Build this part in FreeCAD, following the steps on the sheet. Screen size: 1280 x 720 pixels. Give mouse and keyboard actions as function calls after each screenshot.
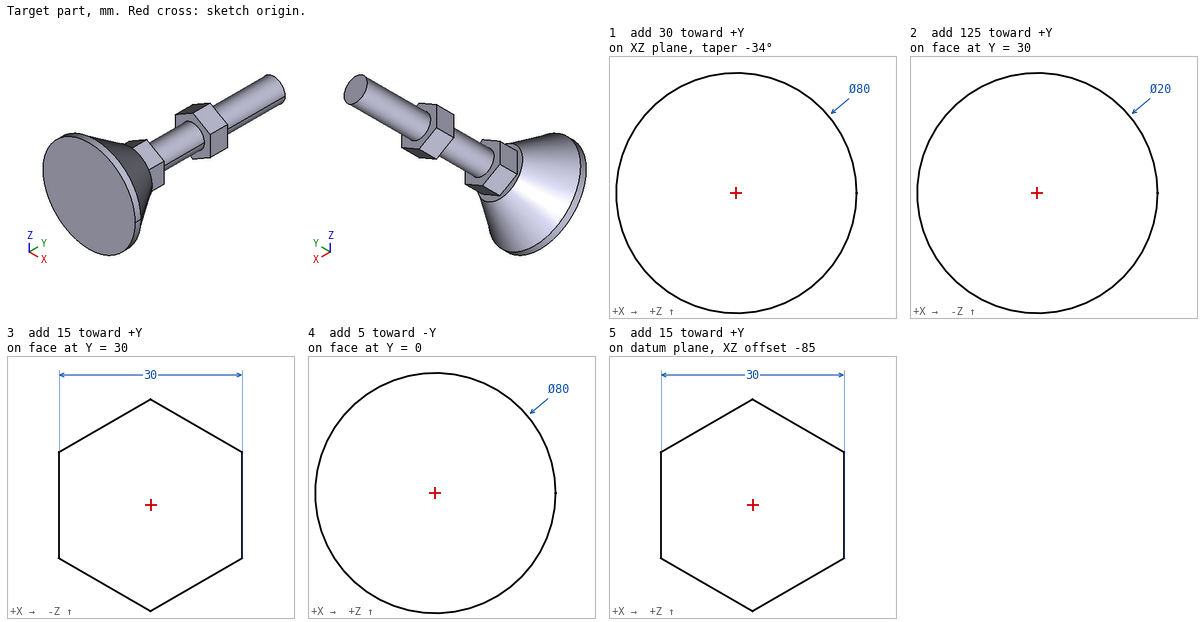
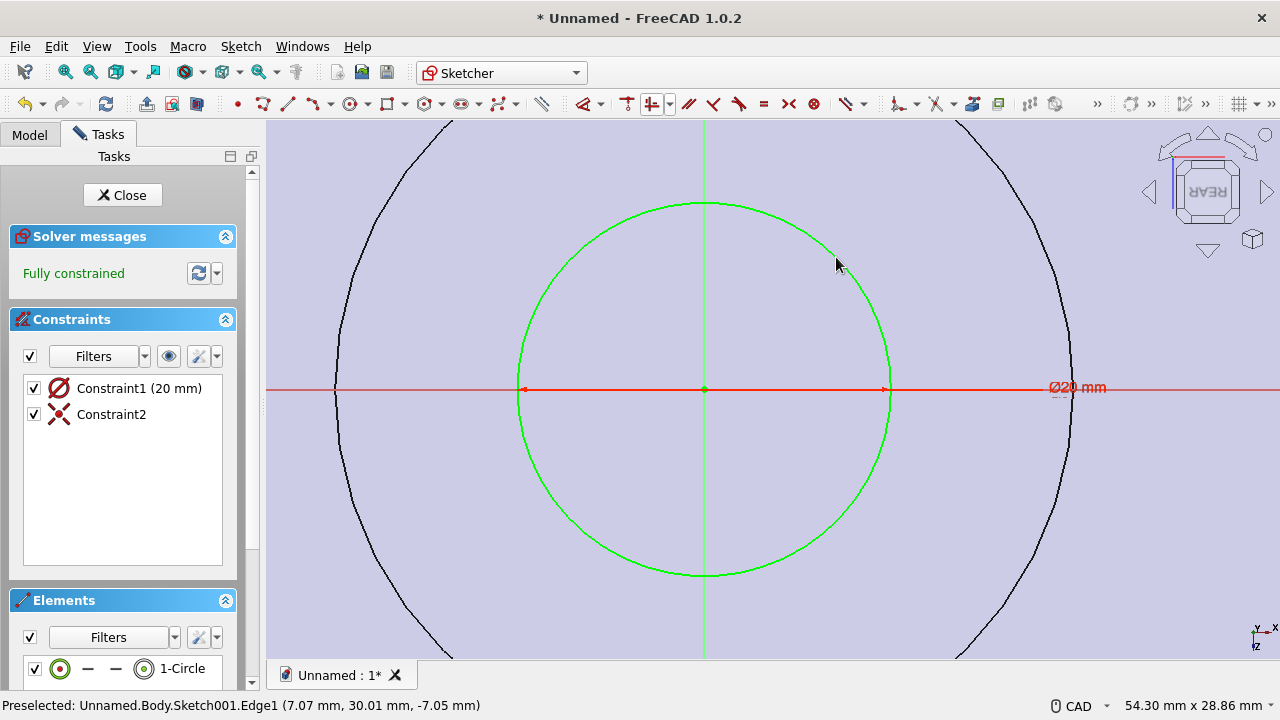
click(123, 195)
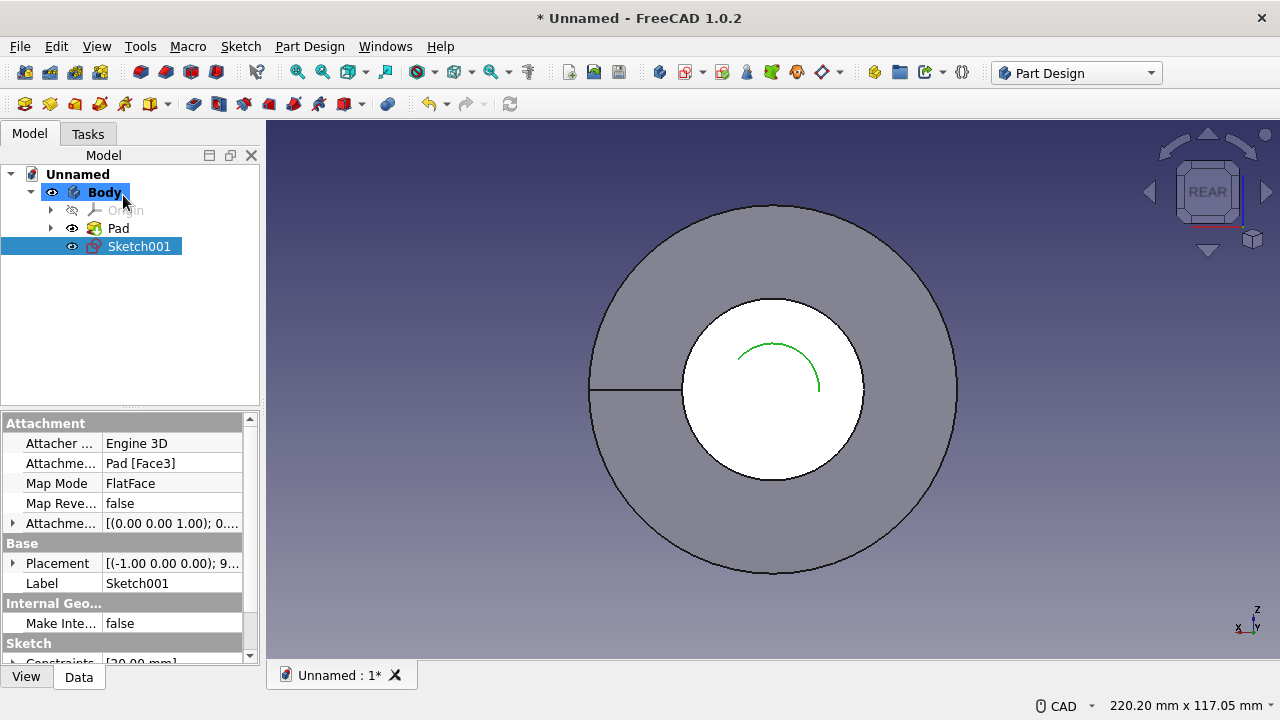
click(25, 104)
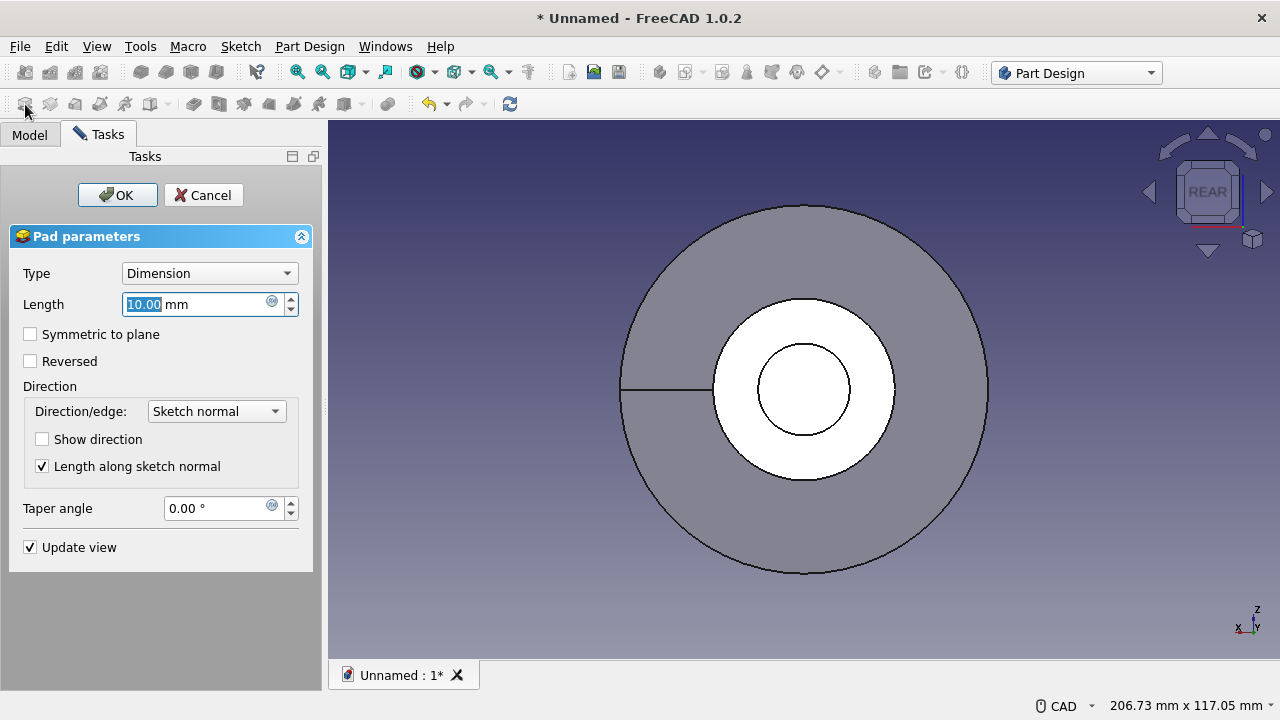
text(125)
key(Tab)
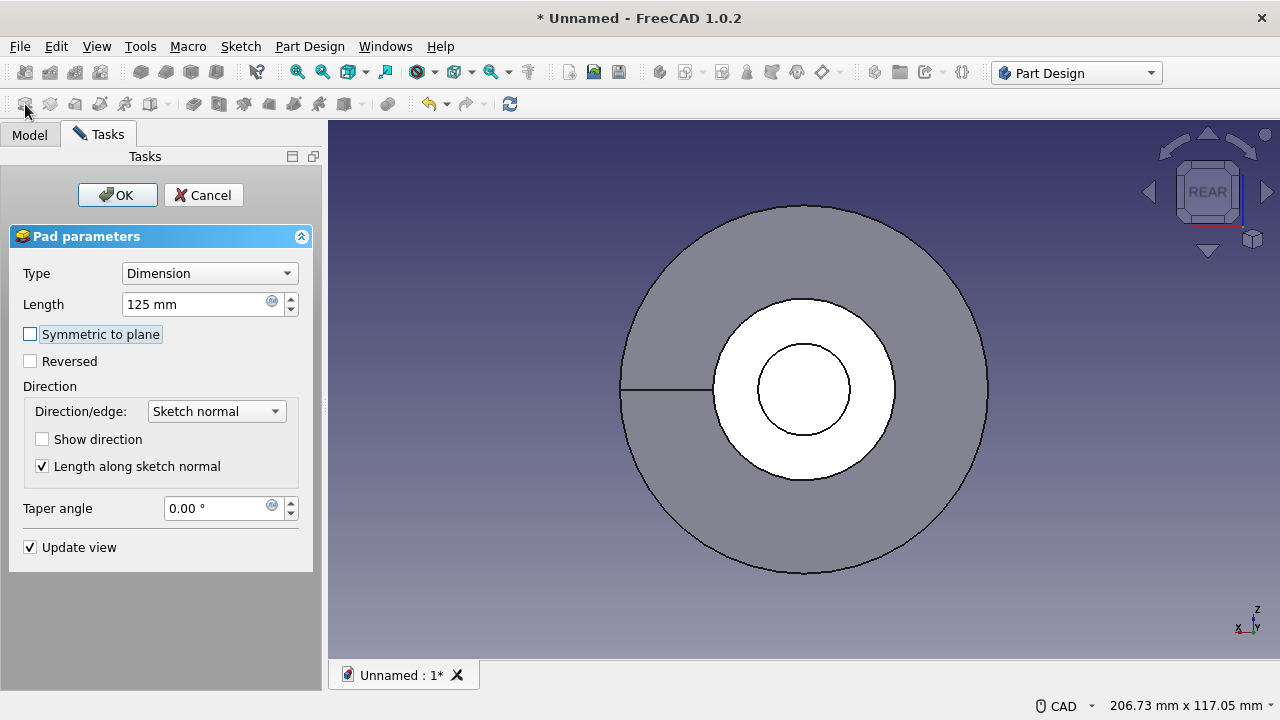
click(118, 195)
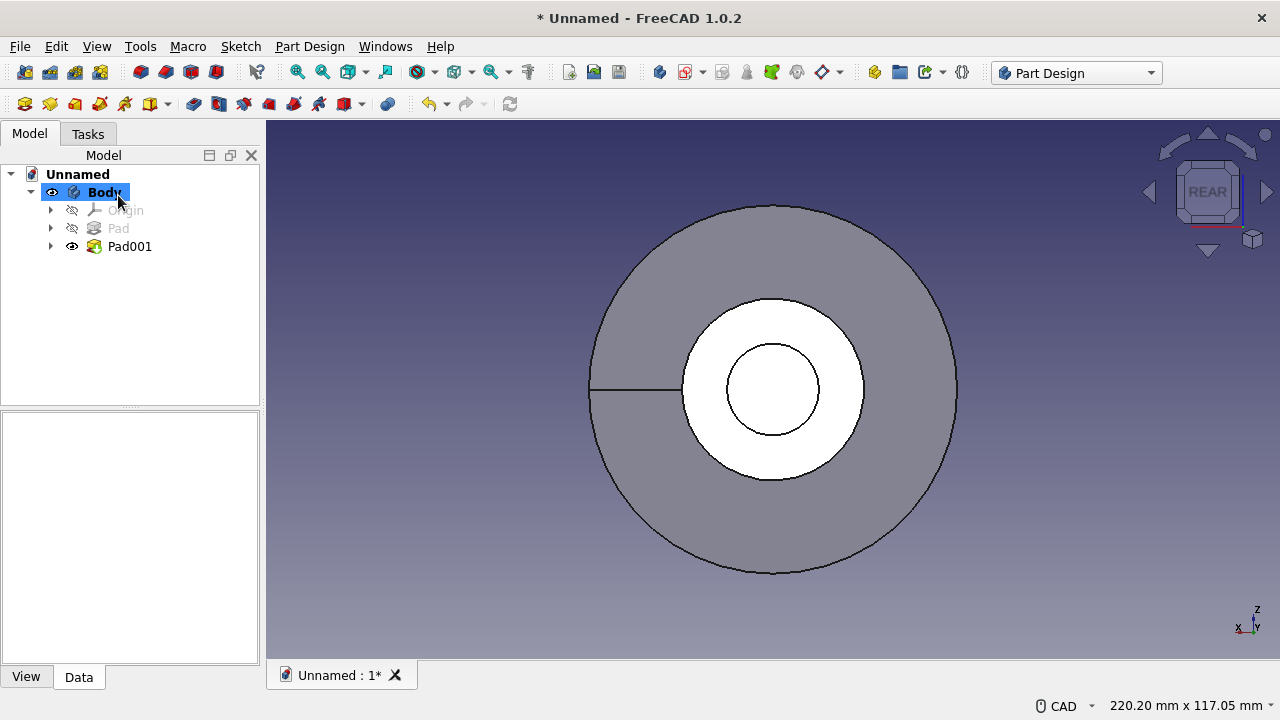
click(721, 336)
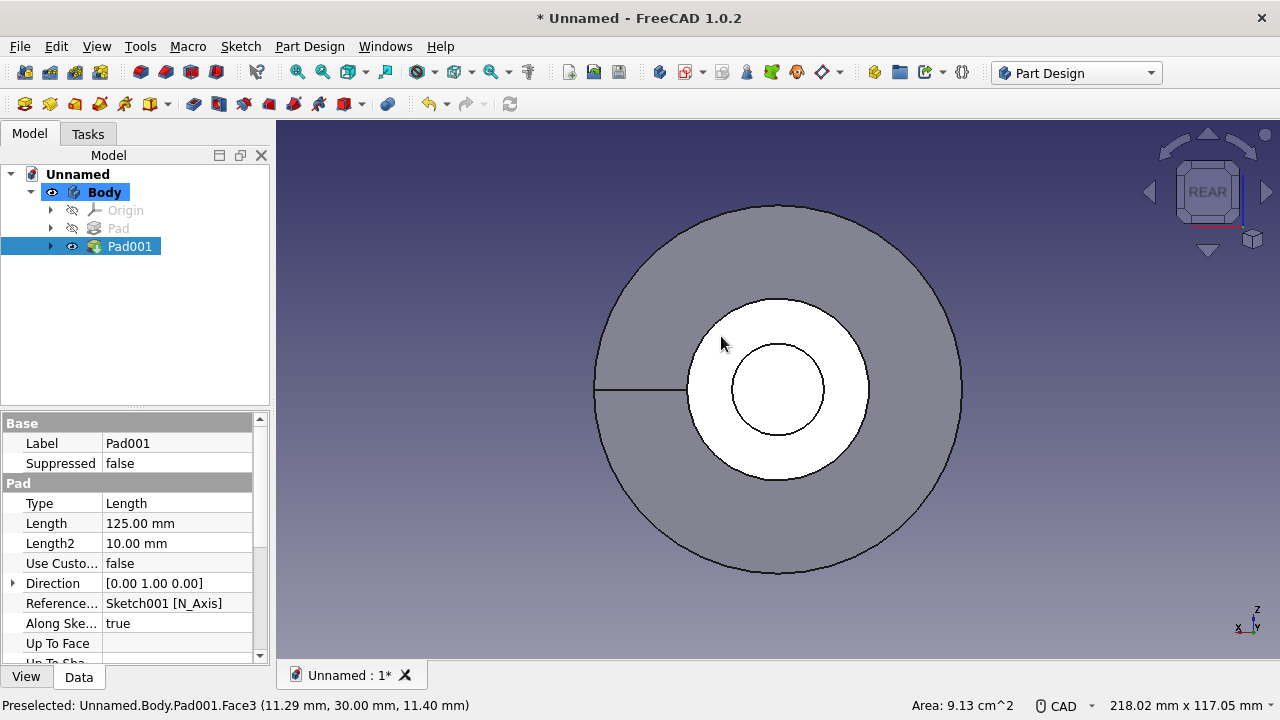
click(684, 72)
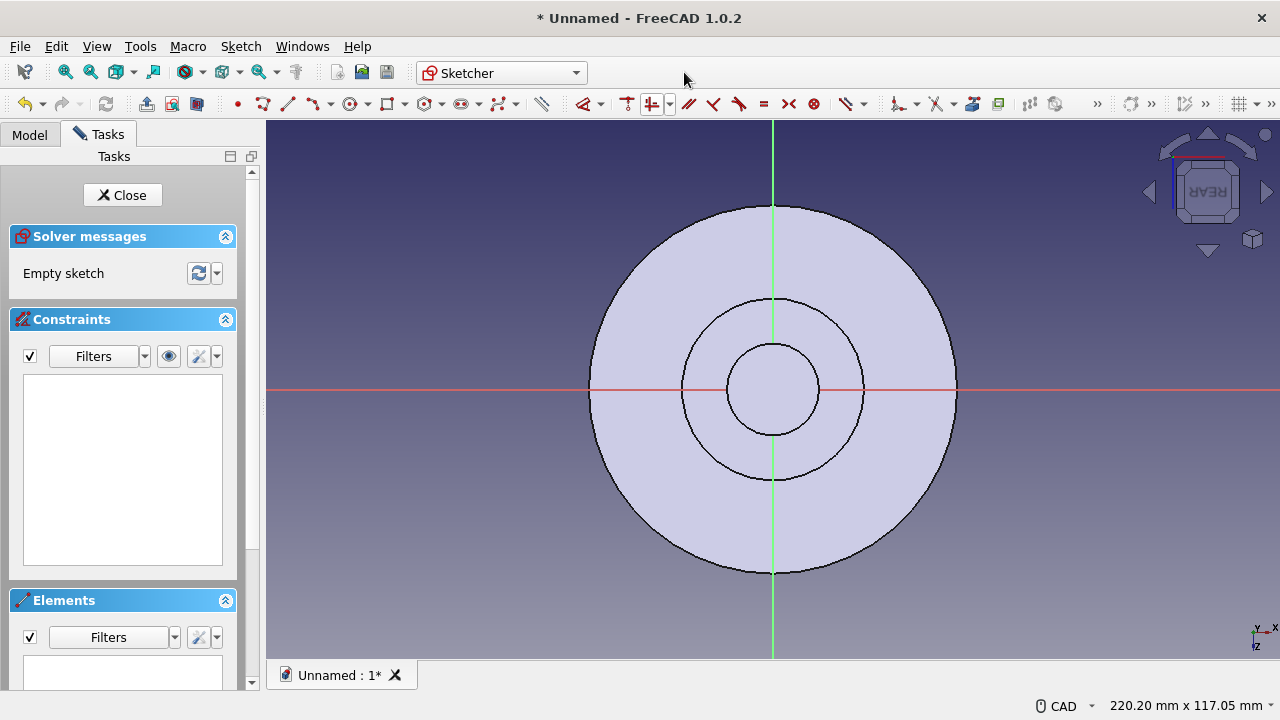
scroll(829, 389, up, 4)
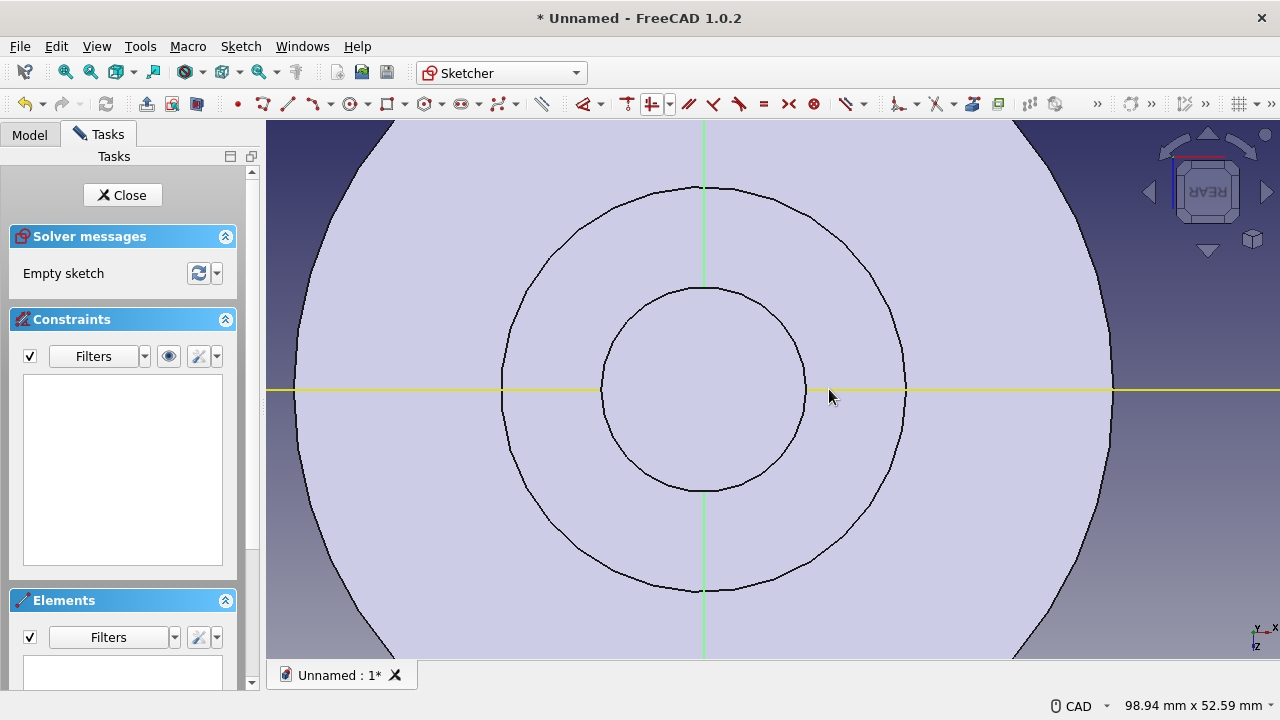
click(424, 104)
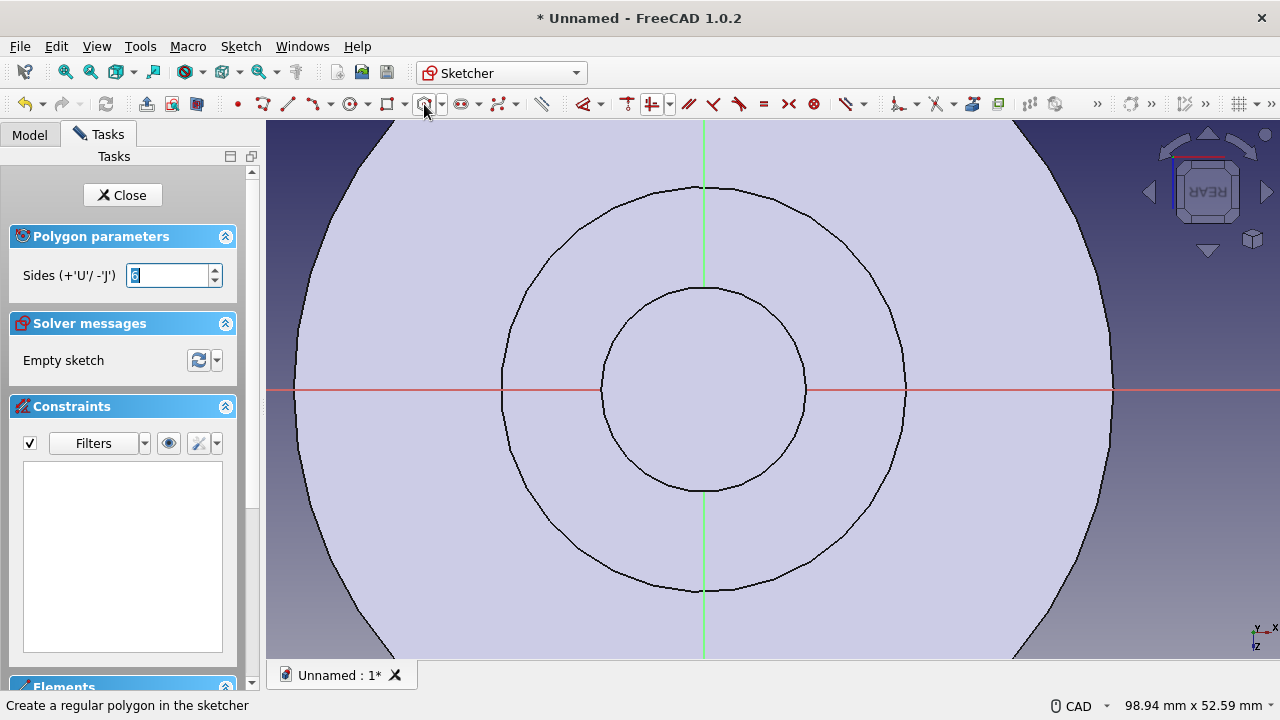
click(704, 389)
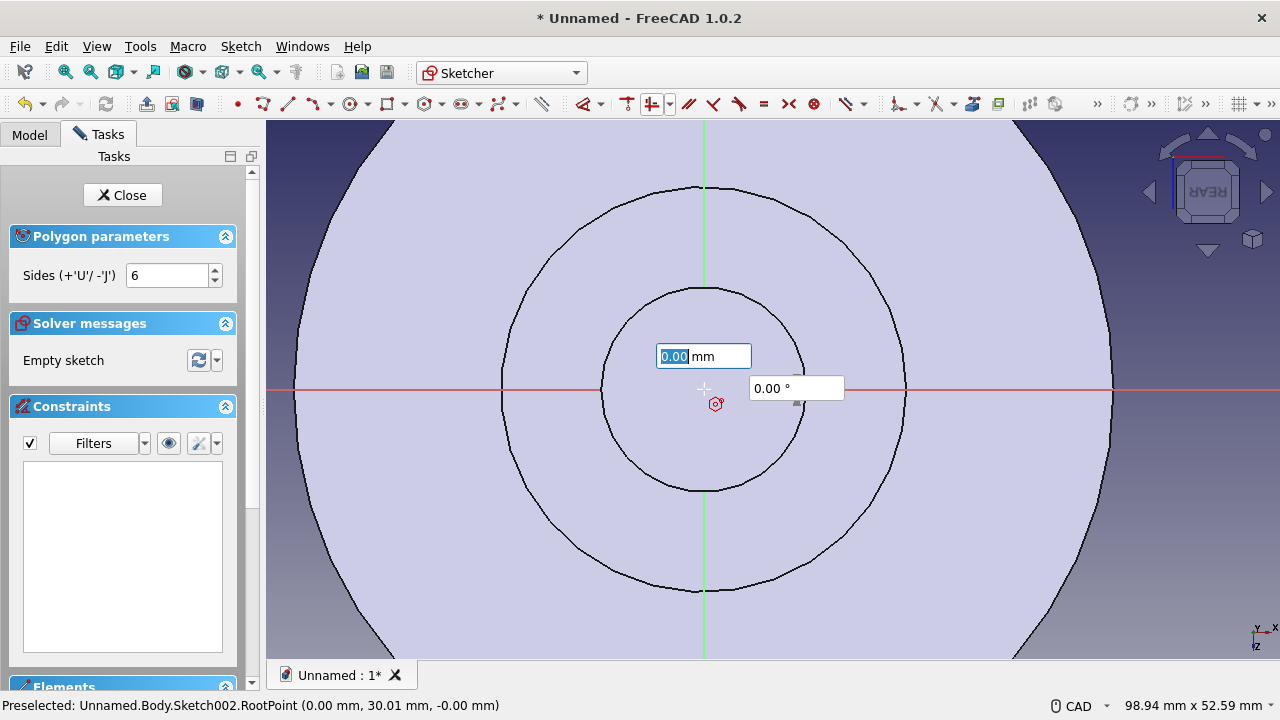
click(704, 212)
right_click(704, 212)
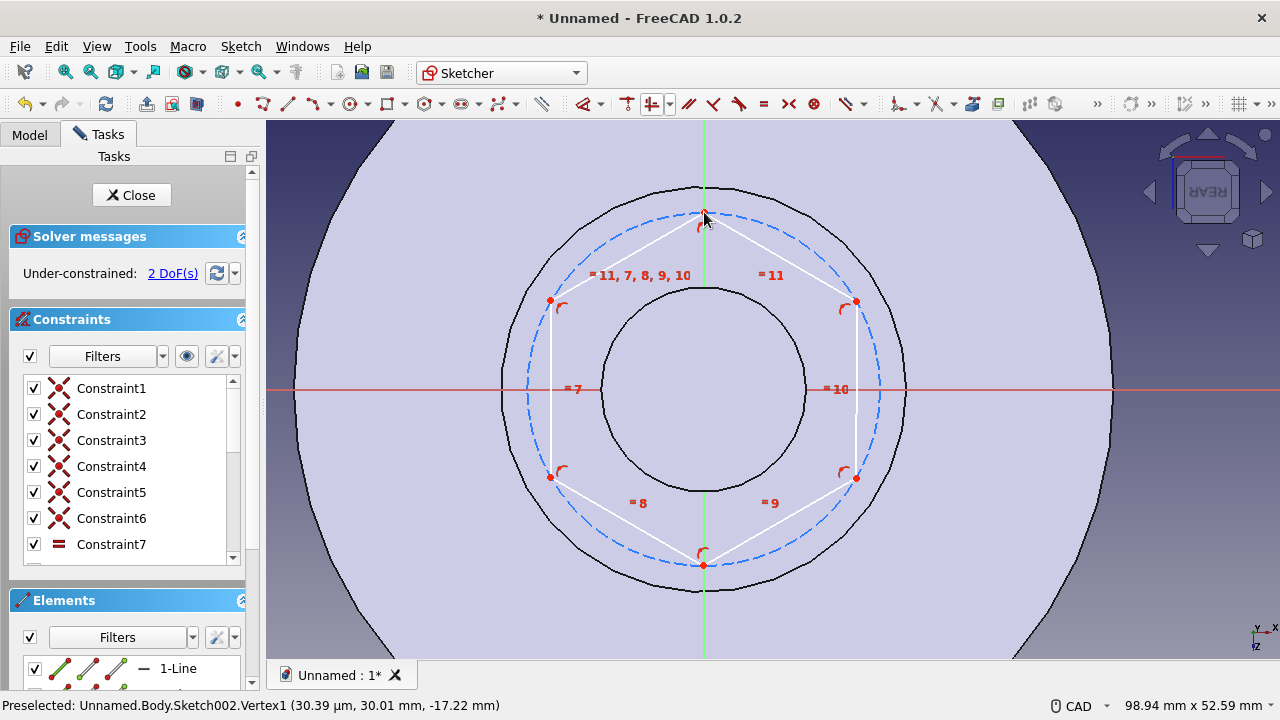
click(551, 354)